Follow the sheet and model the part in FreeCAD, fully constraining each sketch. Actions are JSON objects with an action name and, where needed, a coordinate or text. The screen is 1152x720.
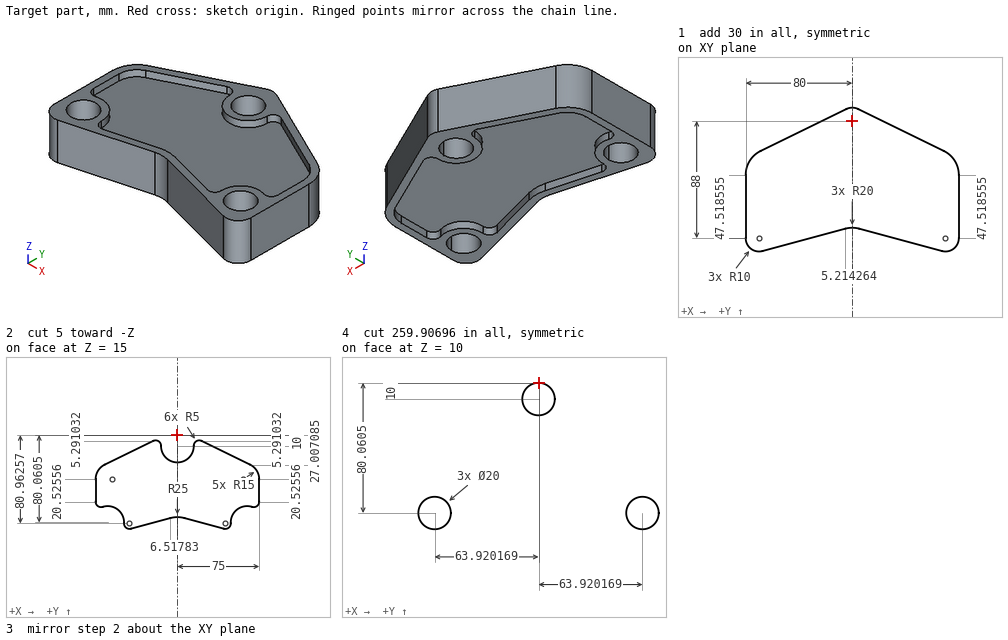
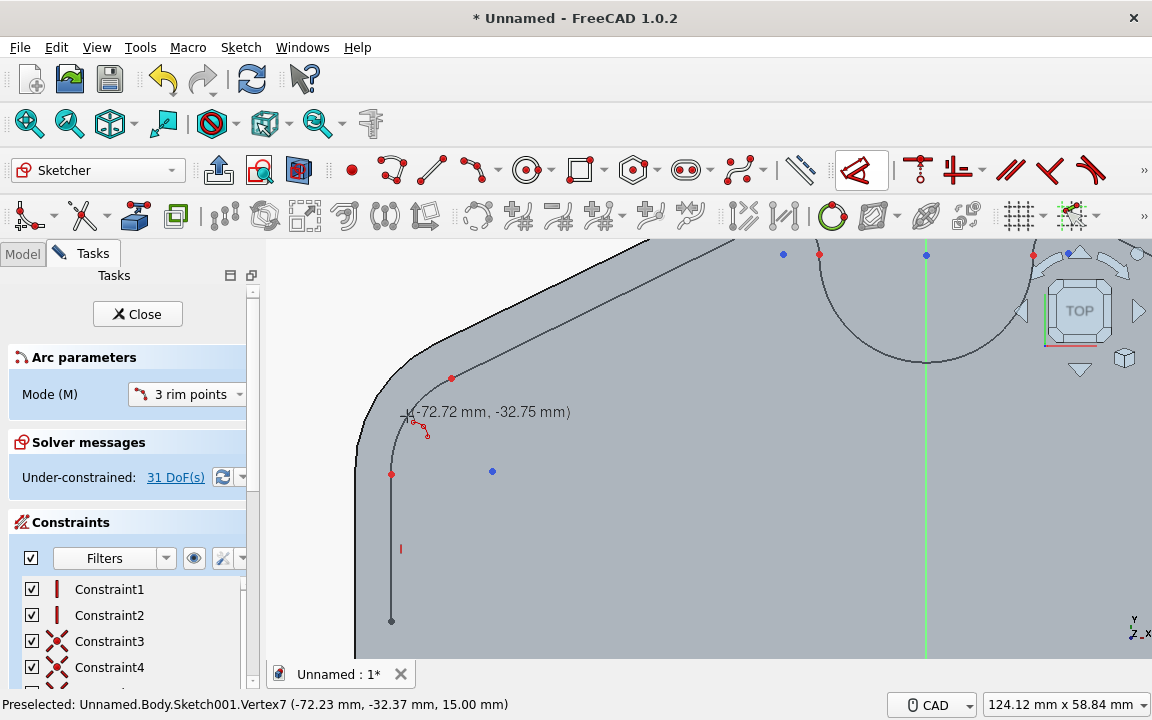
{"action": "left_click", "coordinate": [391, 621]}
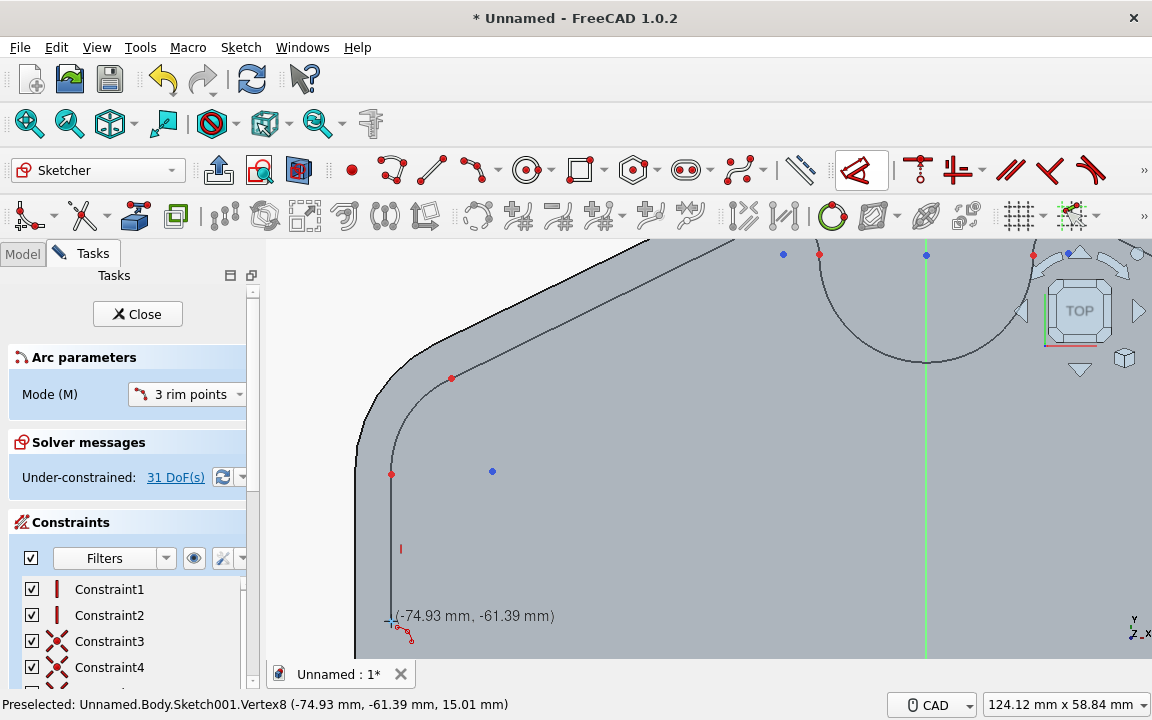
{"action": "scroll", "coordinate": [407, 416], "scroll_direction": "down", "scroll_amount": 4}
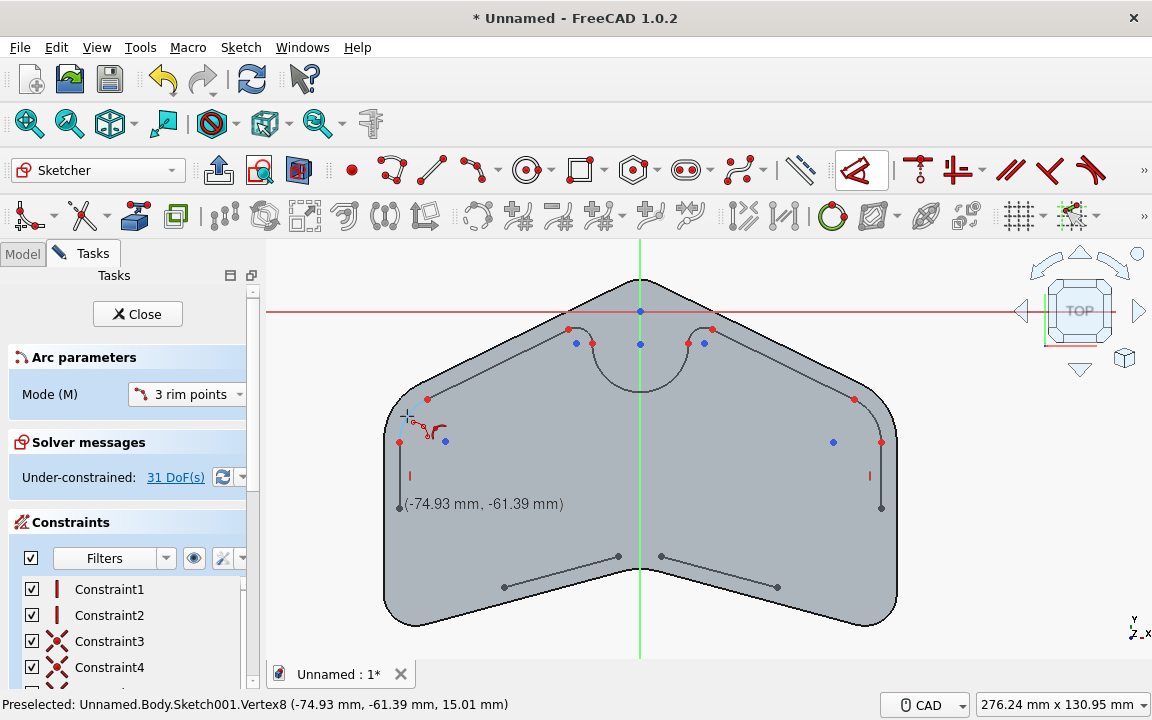
{"action": "left_click", "coordinate": [421, 523]}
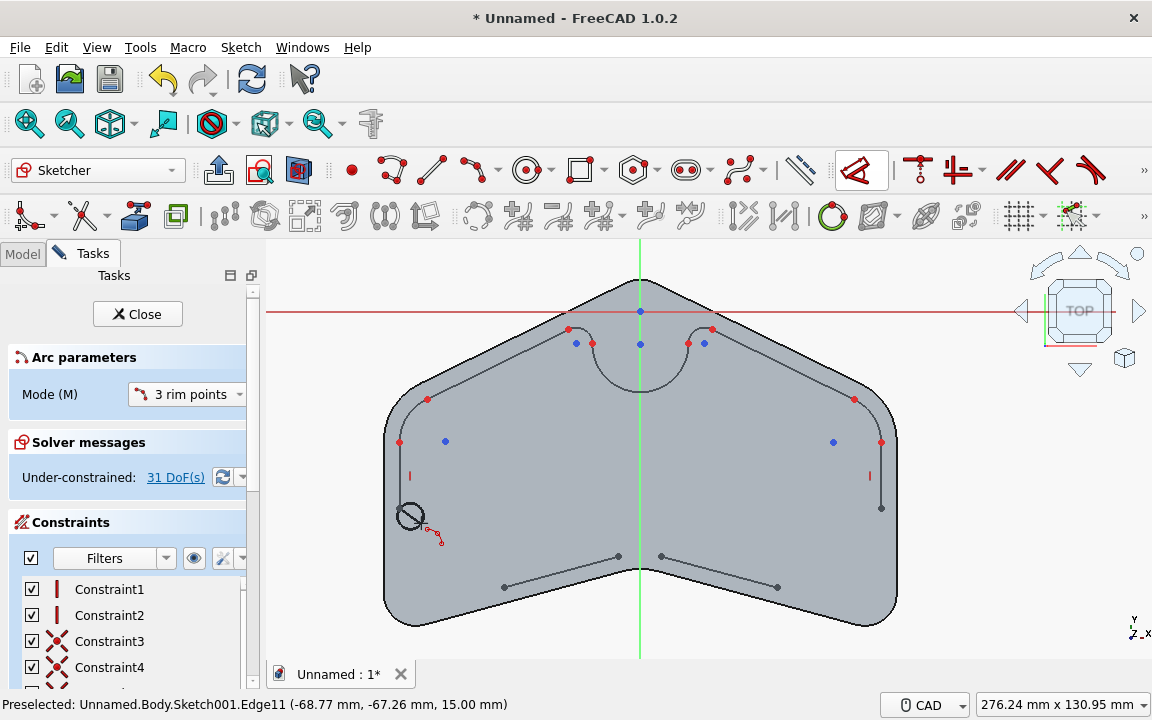
{"action": "scroll", "coordinate": [406, 520], "scroll_direction": "up", "scroll_amount": 5}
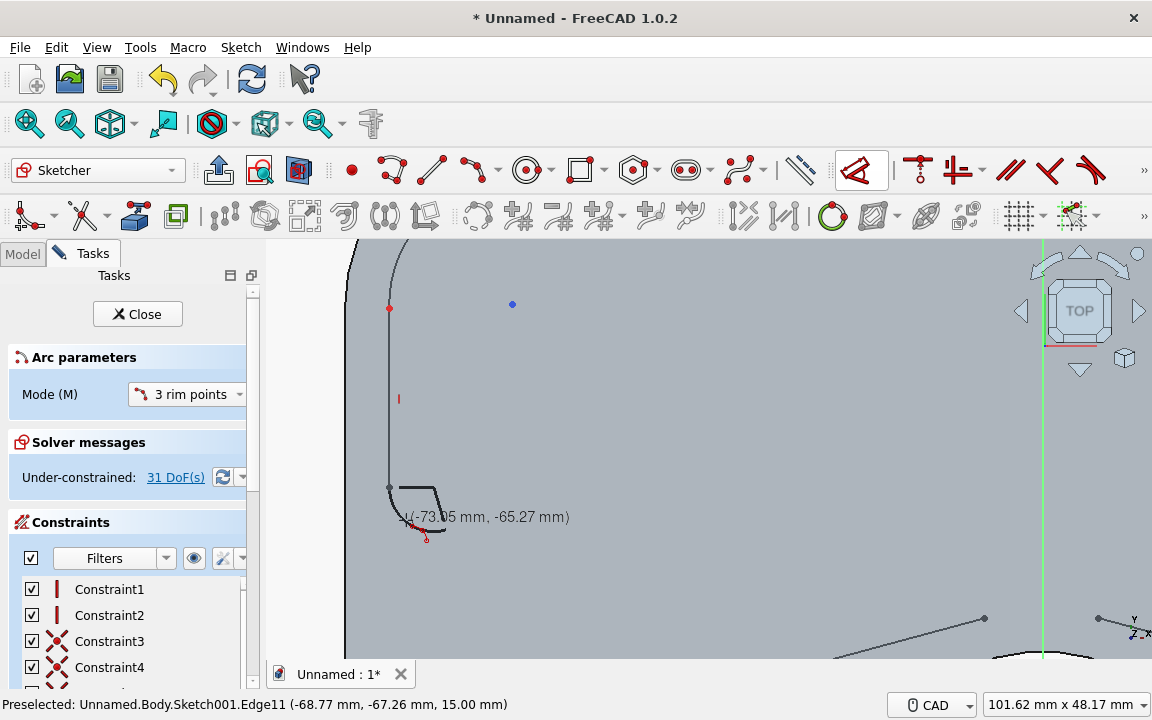
{"action": "left_click", "coordinate": [407, 520]}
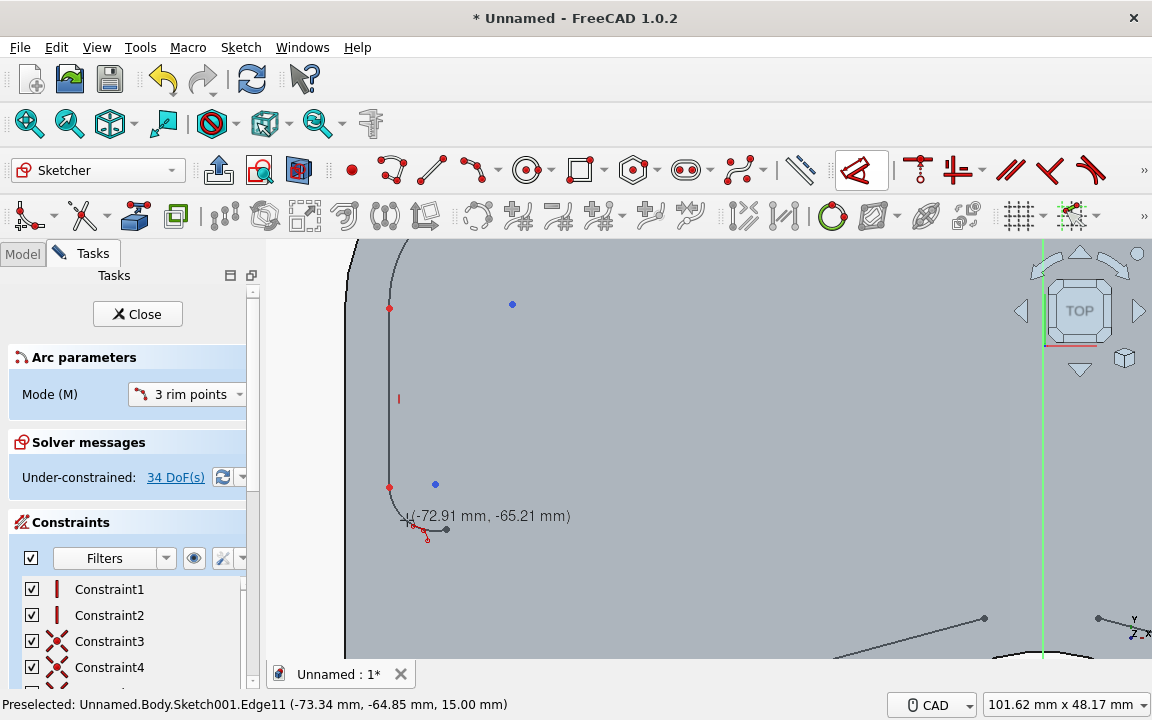
{"action": "left_click", "coordinate": [447, 530]}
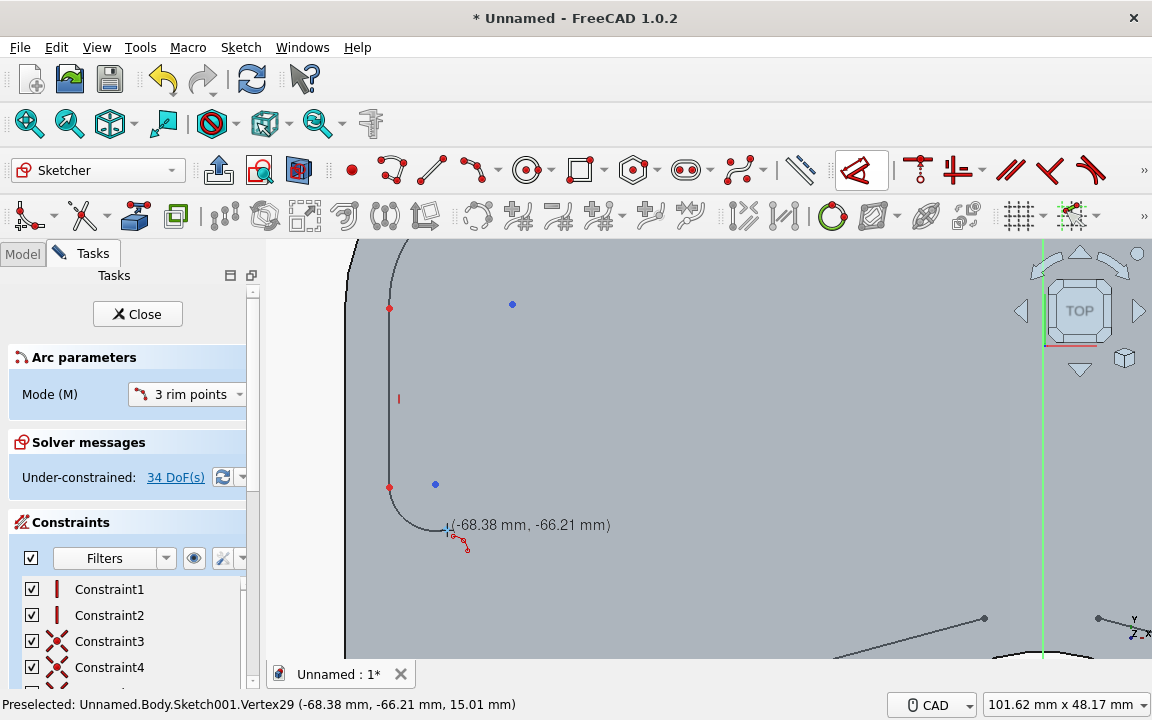
{"action": "scroll", "coordinate": [406, 520], "scroll_direction": "down", "scroll_amount": 5}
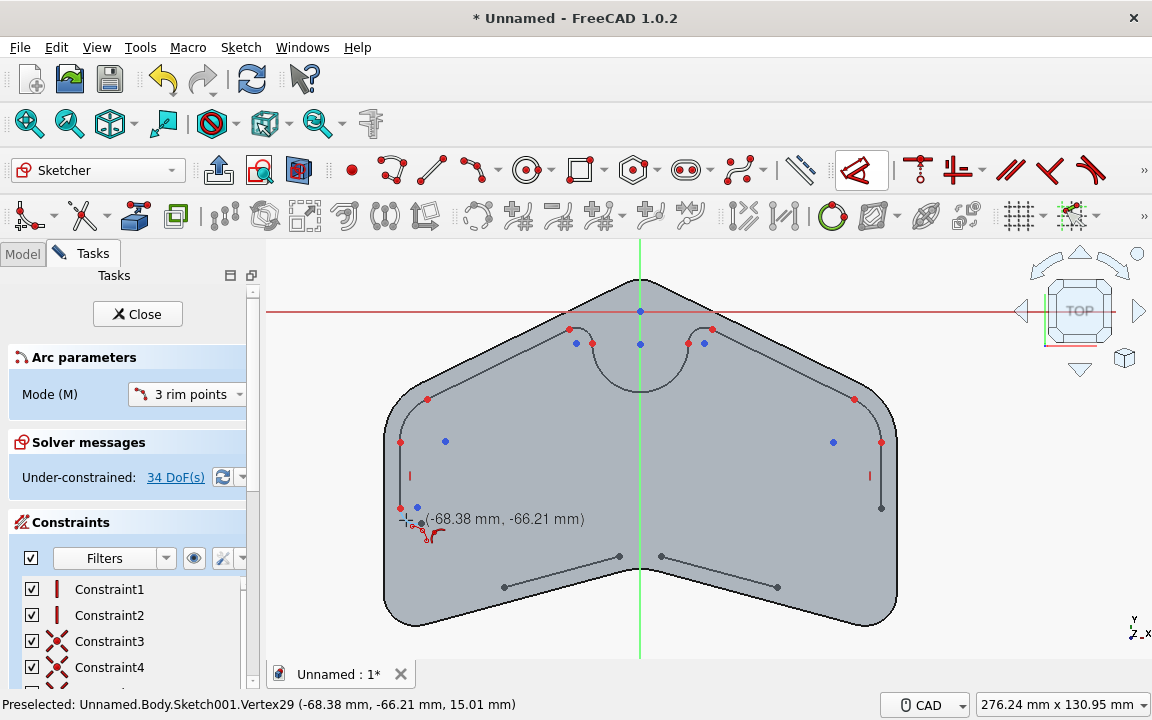
{"action": "left_click", "coordinate": [483, 571]}
{"action": "left_click", "coordinate": [465, 530]}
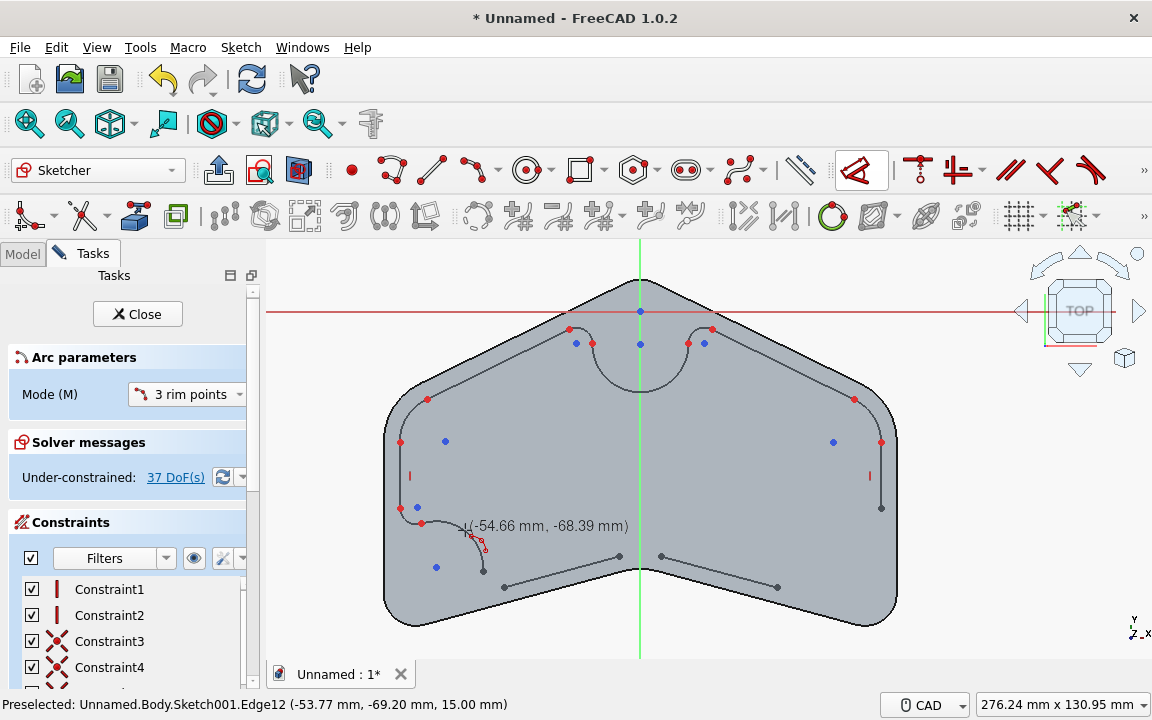
{"action": "left_click", "coordinate": [483, 572]}
{"action": "left_click", "coordinate": [504, 588]}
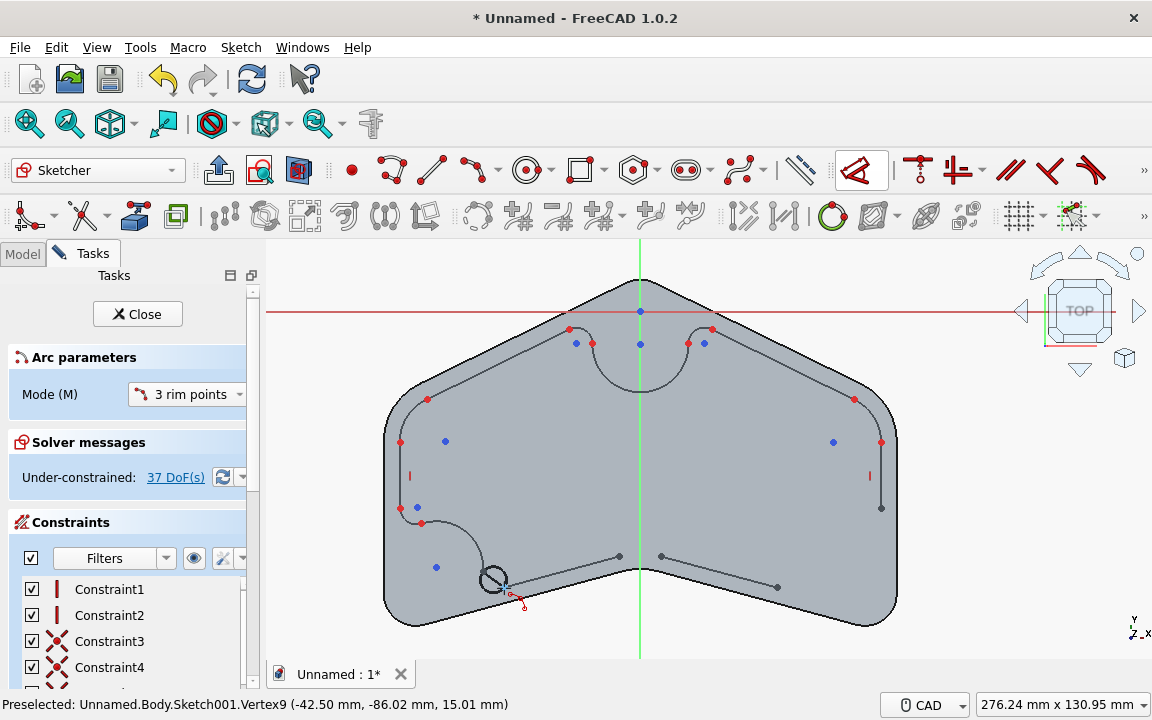
{"action": "scroll", "coordinate": [489, 584], "scroll_direction": "up", "scroll_amount": 5}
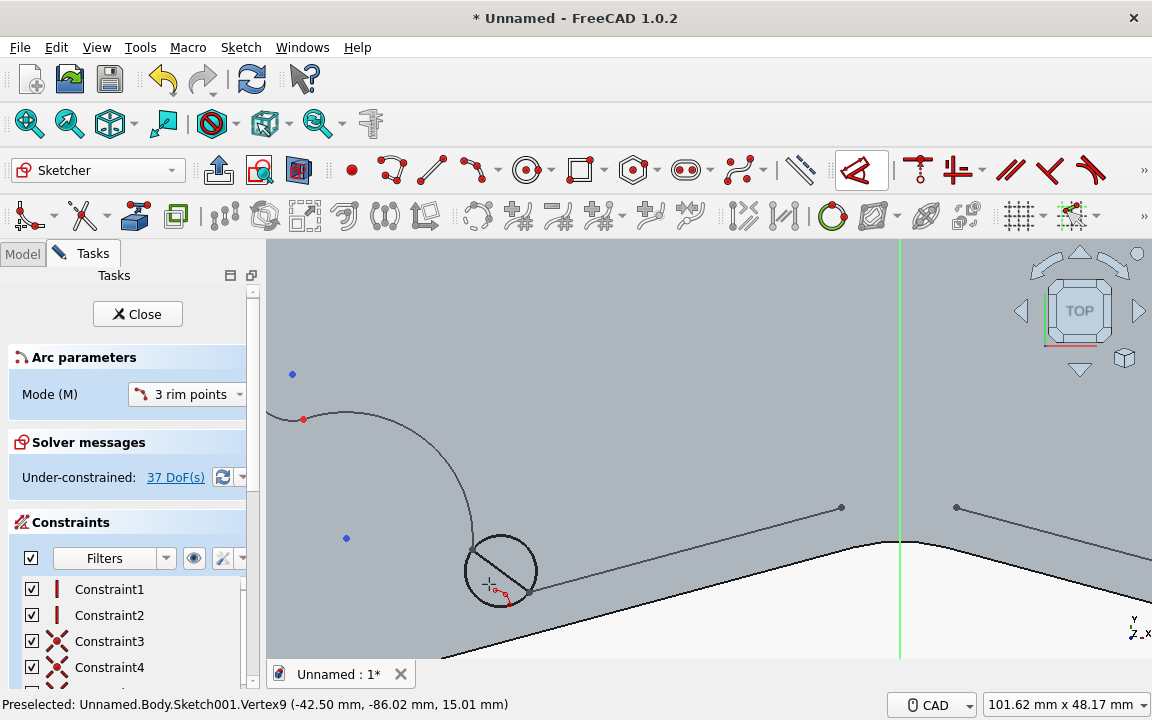
{"action": "left_click", "coordinate": [490, 582]}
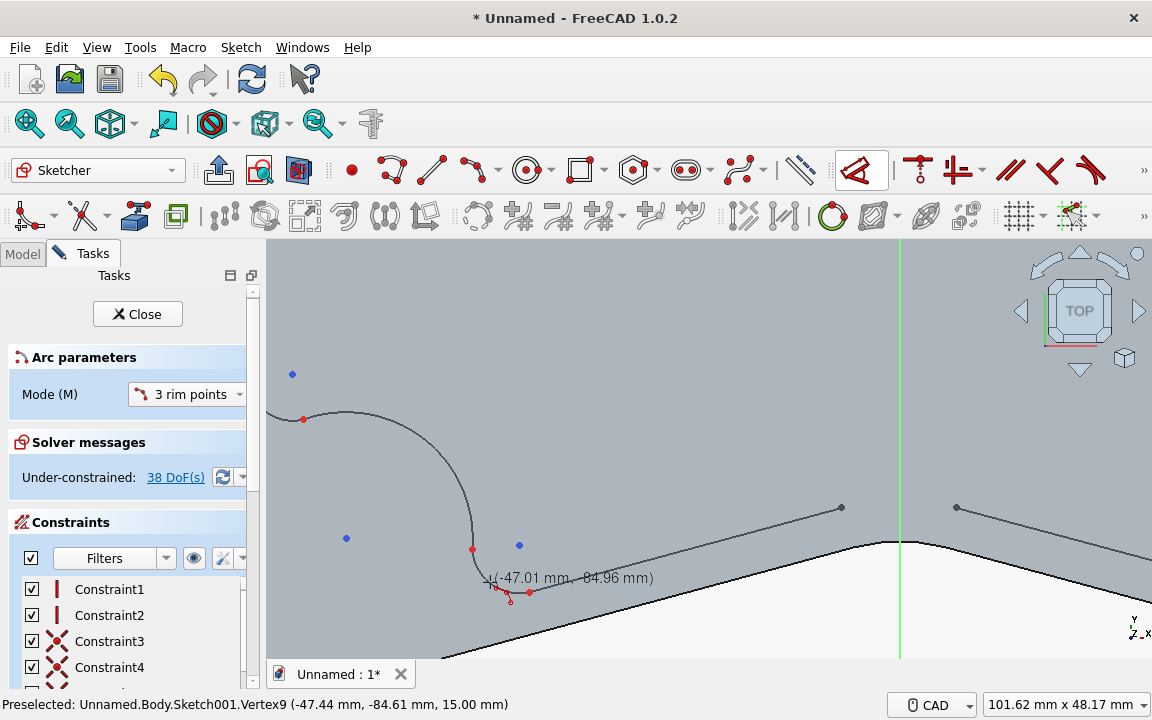
{"action": "left_click", "coordinate": [842, 508]}
{"action": "left_click", "coordinate": [956, 508]}